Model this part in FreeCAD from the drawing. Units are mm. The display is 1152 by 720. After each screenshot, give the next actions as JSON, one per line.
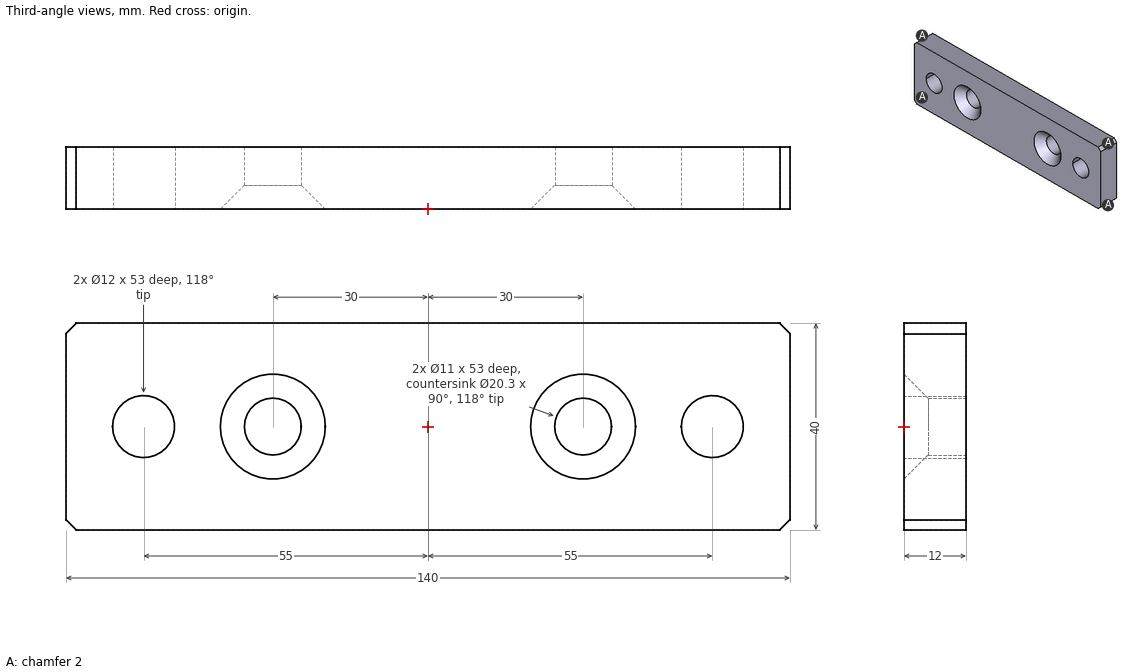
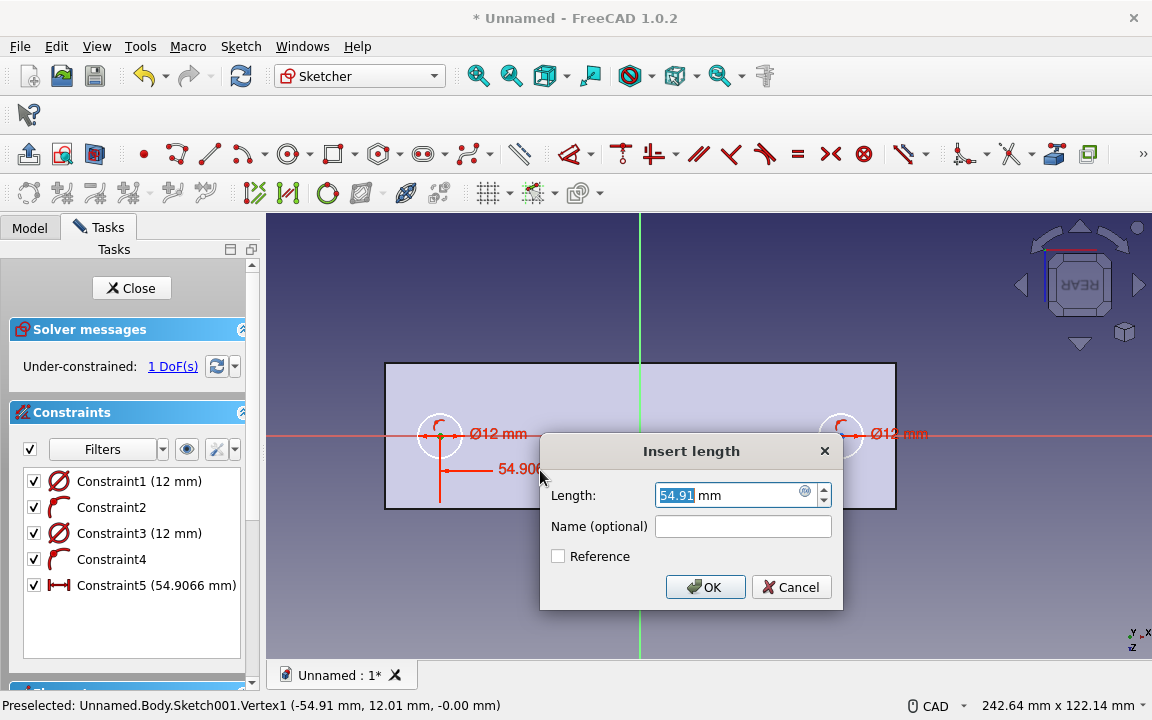
{"action": "type", "text": "55"}
{"action": "key", "text": "Return"}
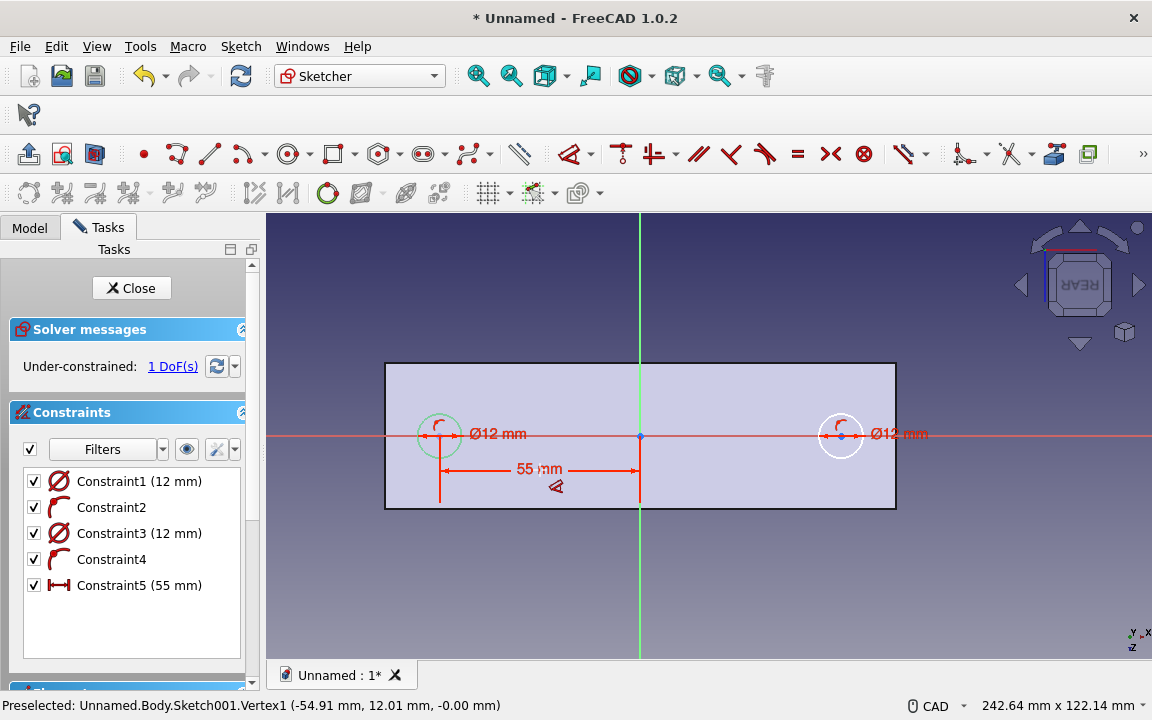
{"action": "left_click", "coordinate": [841, 436]}
{"action": "left_click", "coordinate": [741, 470]}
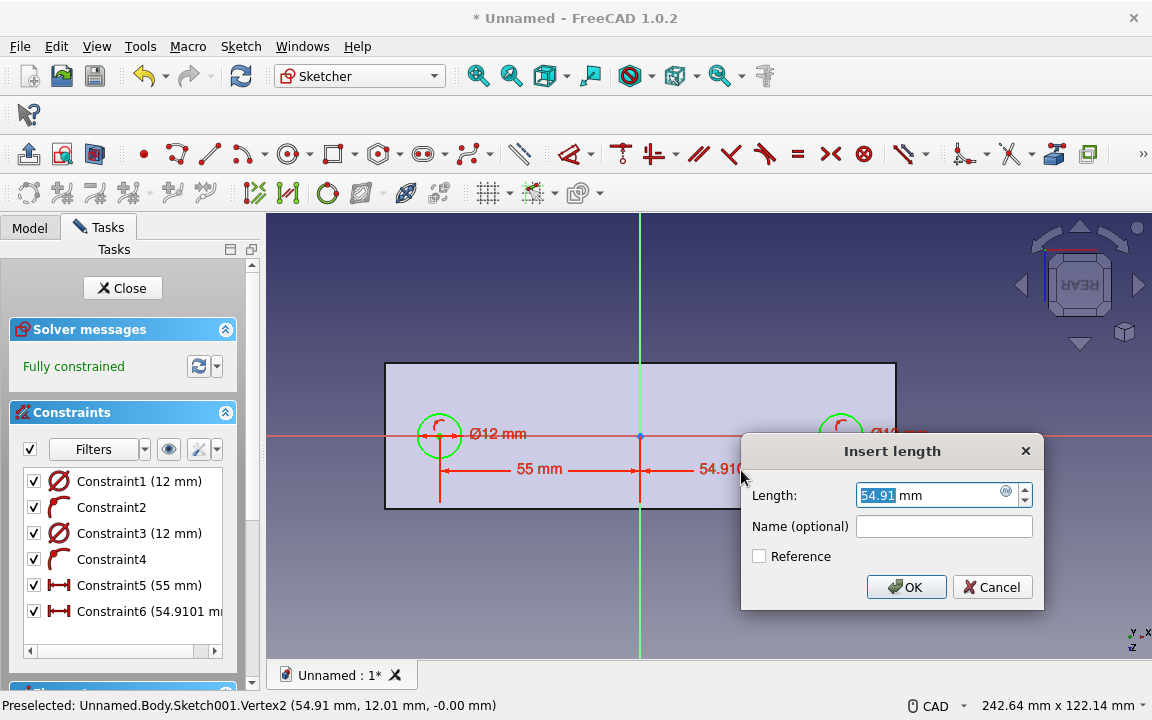
{"action": "type", "text": "55"}
{"action": "key", "text": "Return"}
{"action": "key", "text": "Escape"}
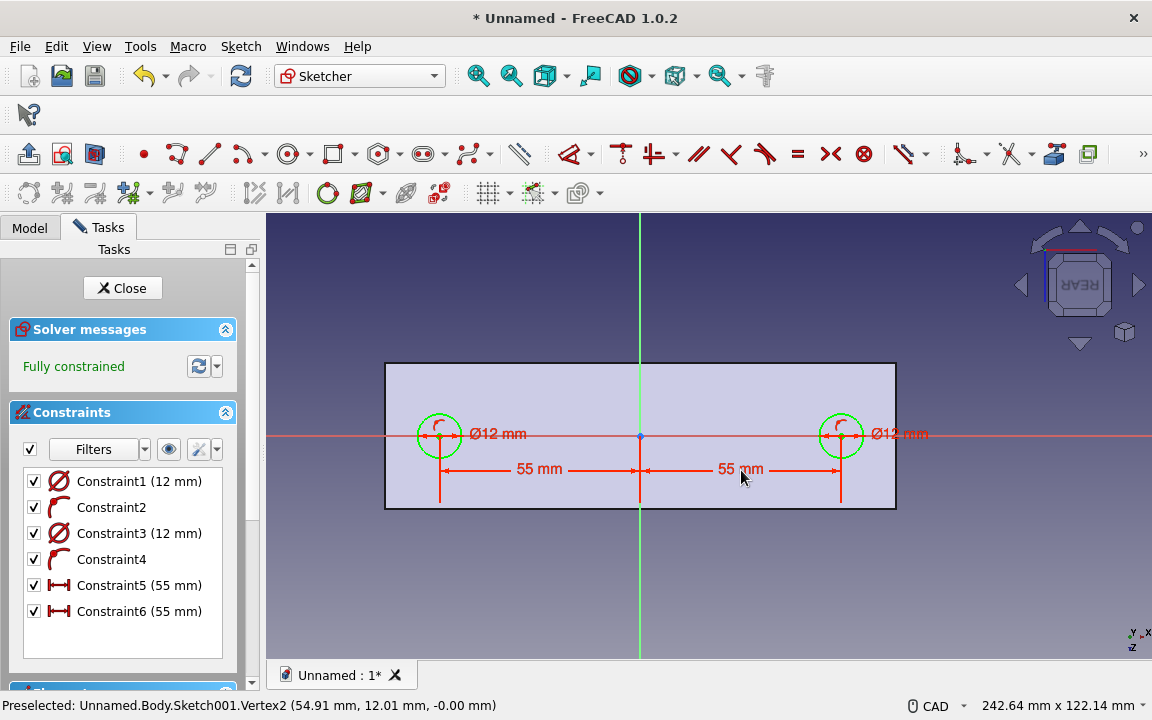
{"action": "left_click", "coordinate": [123, 288]}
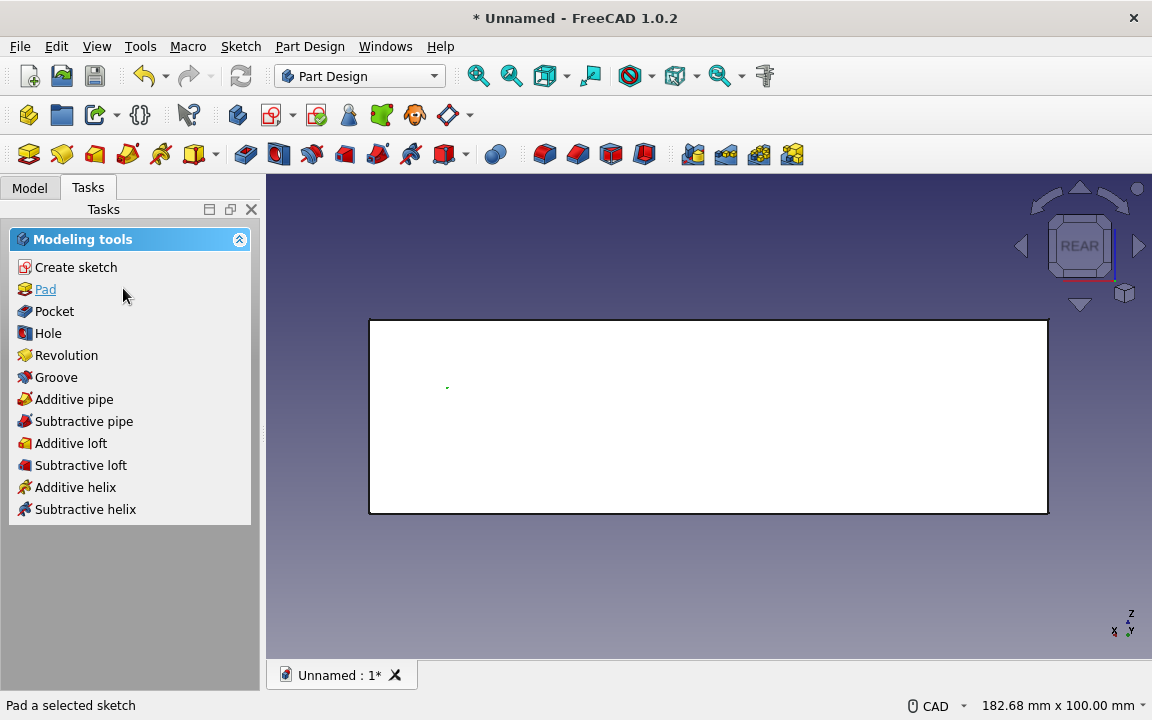
{"action": "left_click", "coordinate": [279, 154]}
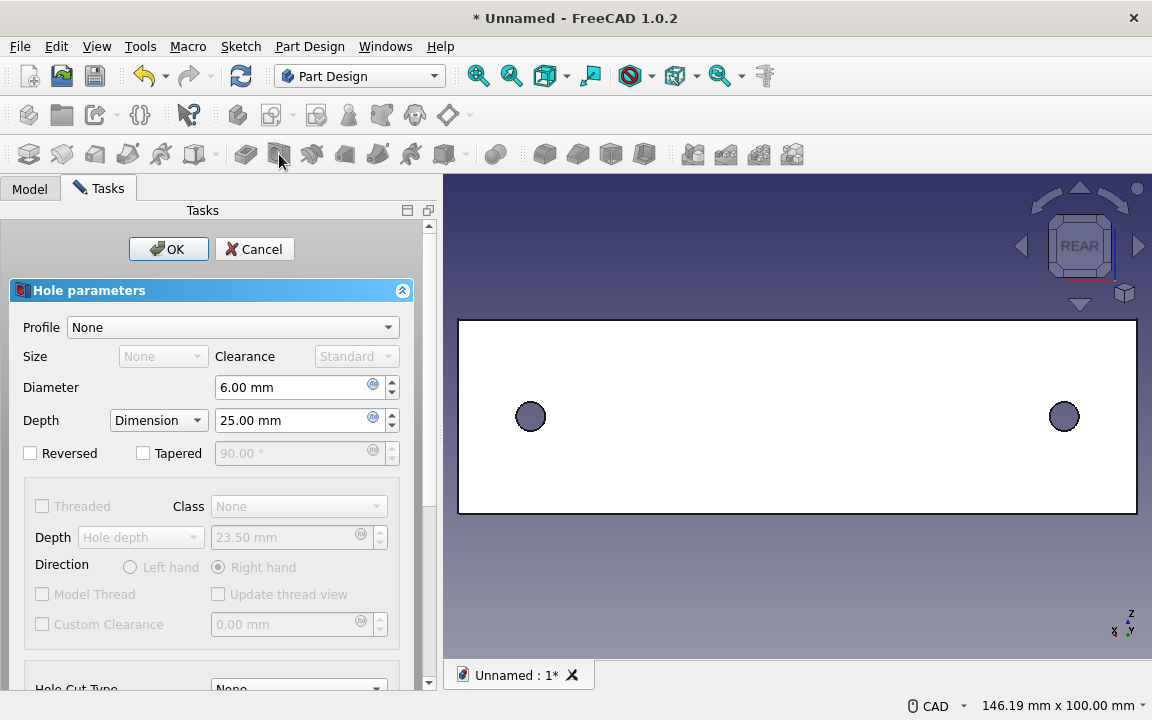
{"action": "triple_click", "coordinate": [300, 388]}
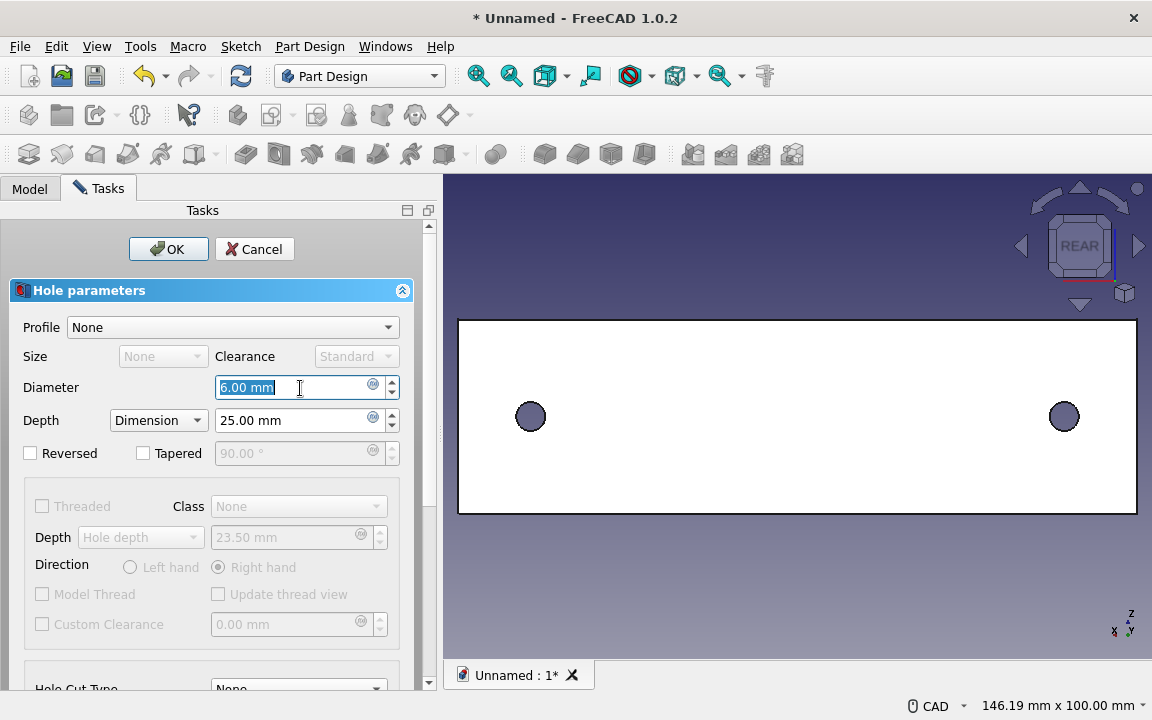
{"action": "type", "text": "12"}
{"action": "key", "text": "Tab"}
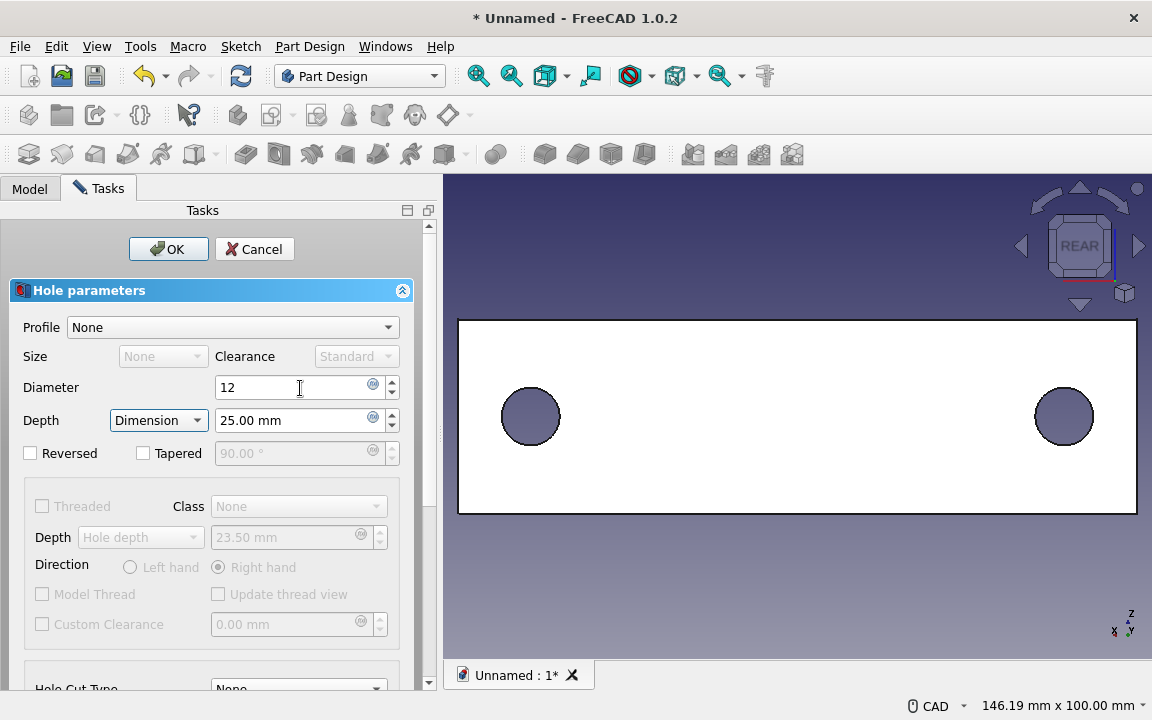
{"action": "triple_click", "coordinate": [300, 420]}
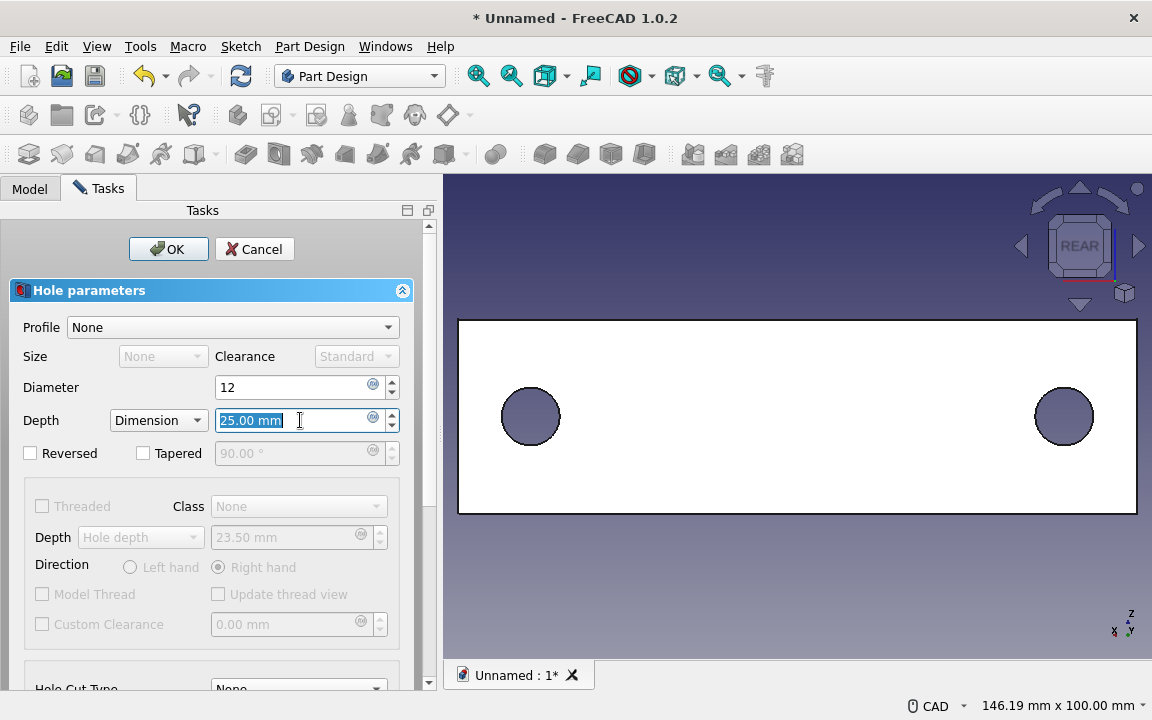
{"action": "type", "text": "53"}
{"action": "key", "text": "Tab"}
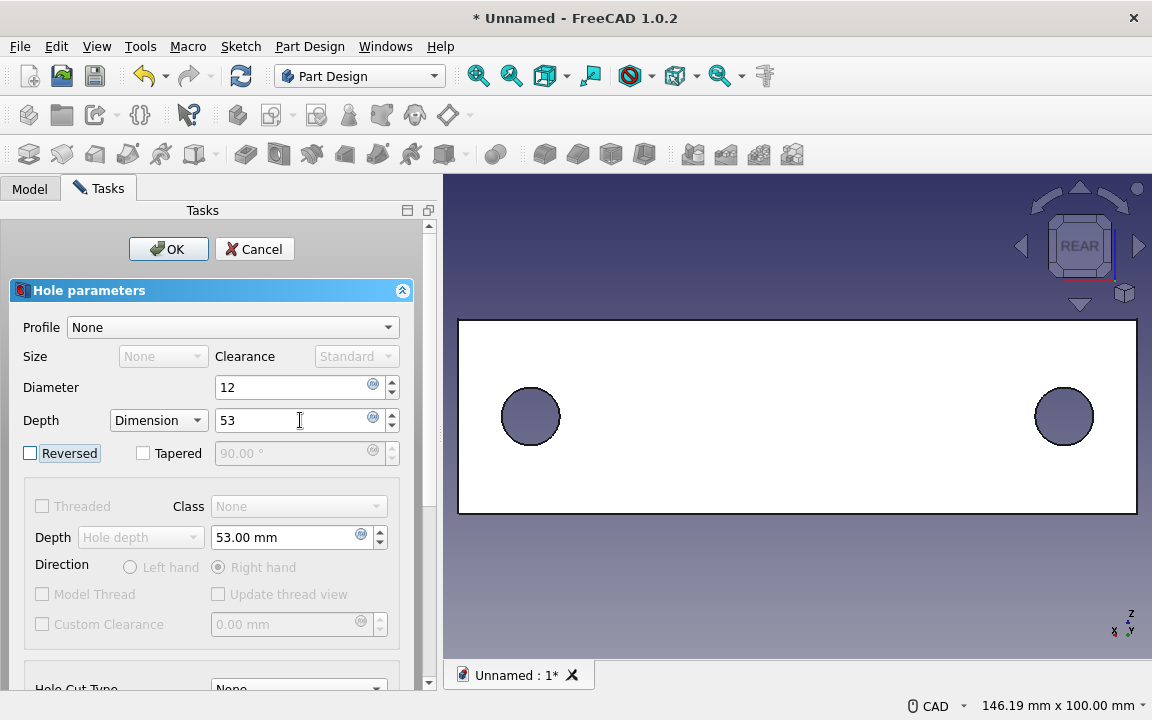
{"action": "left_click", "coordinate": [169, 249]}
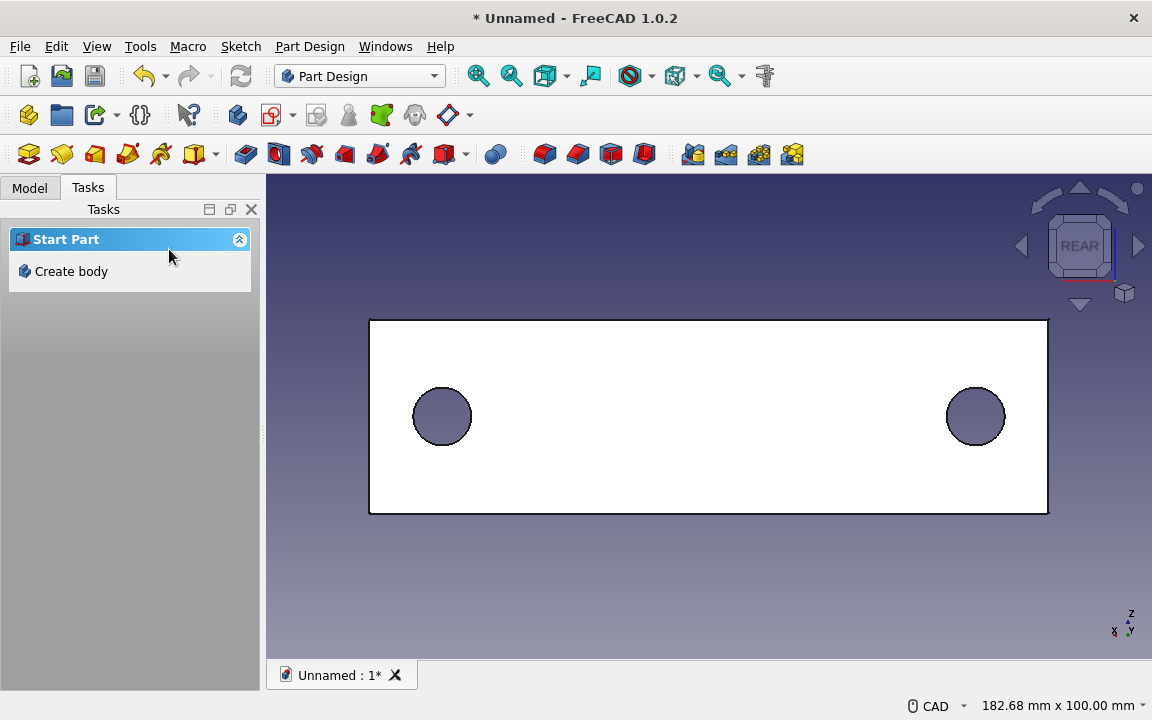
{"action": "key", "text": "0"}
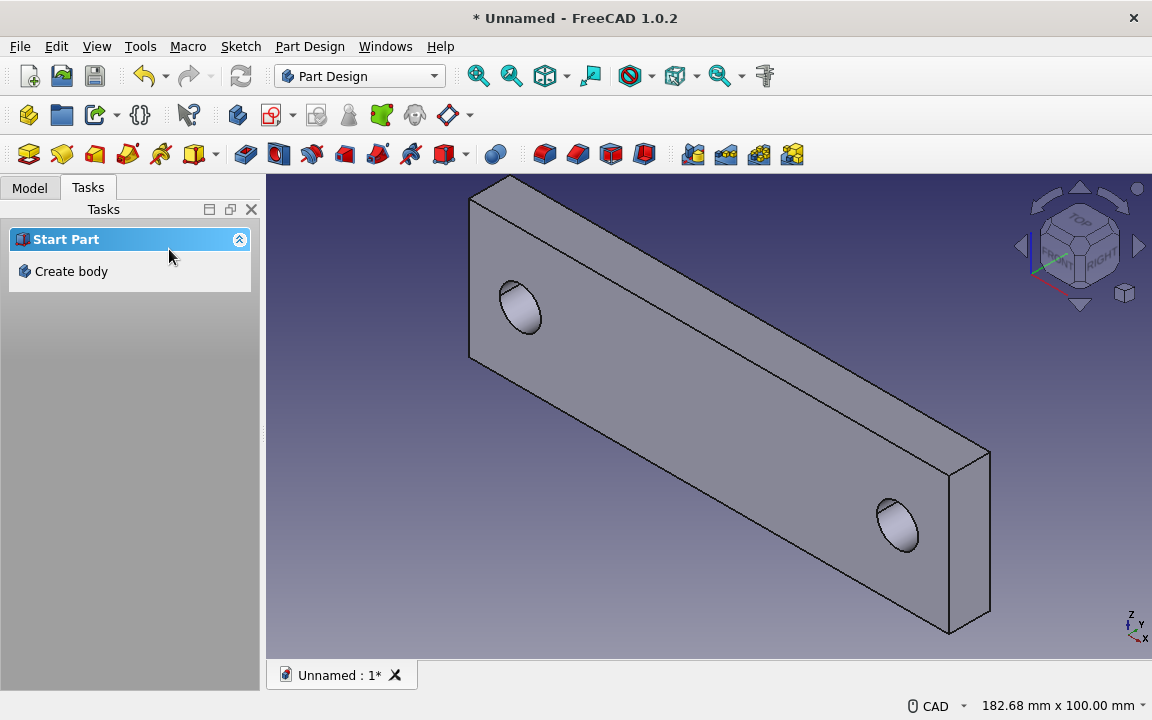
{"action": "left_click", "coordinate": [778, 455]}